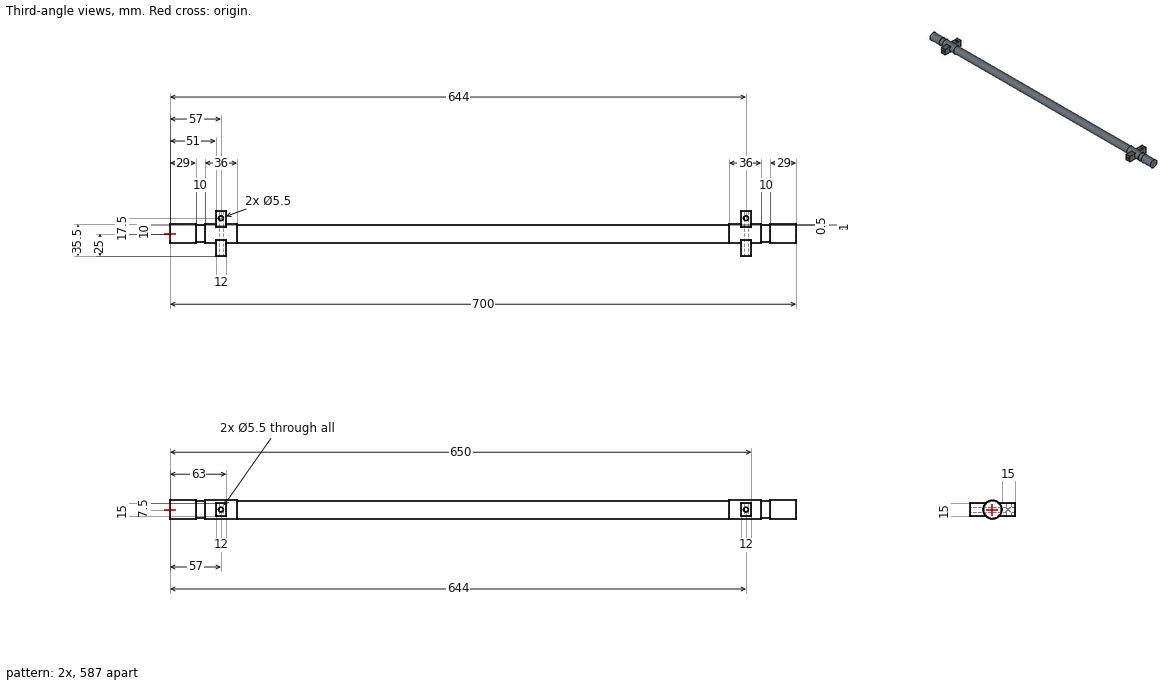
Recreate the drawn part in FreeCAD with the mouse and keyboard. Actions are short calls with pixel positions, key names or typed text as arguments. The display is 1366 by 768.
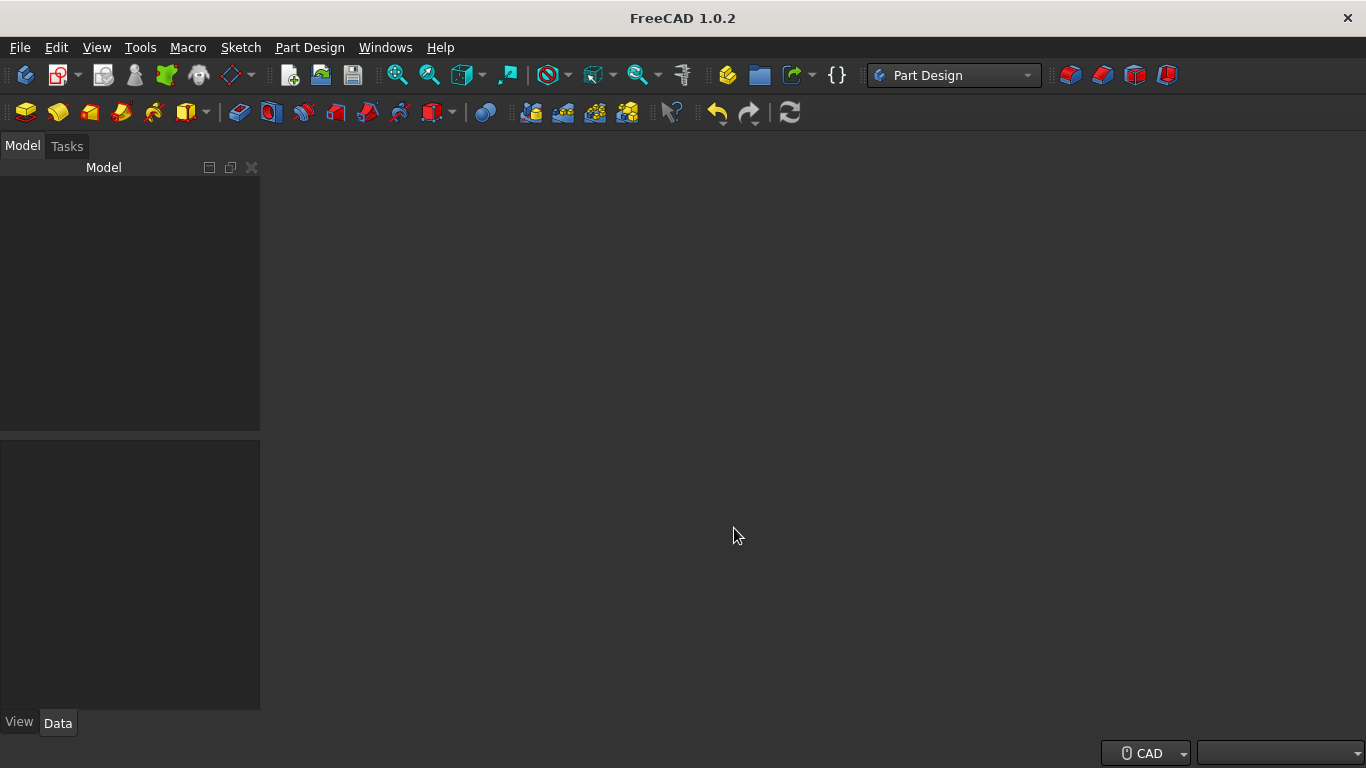
click(290, 76)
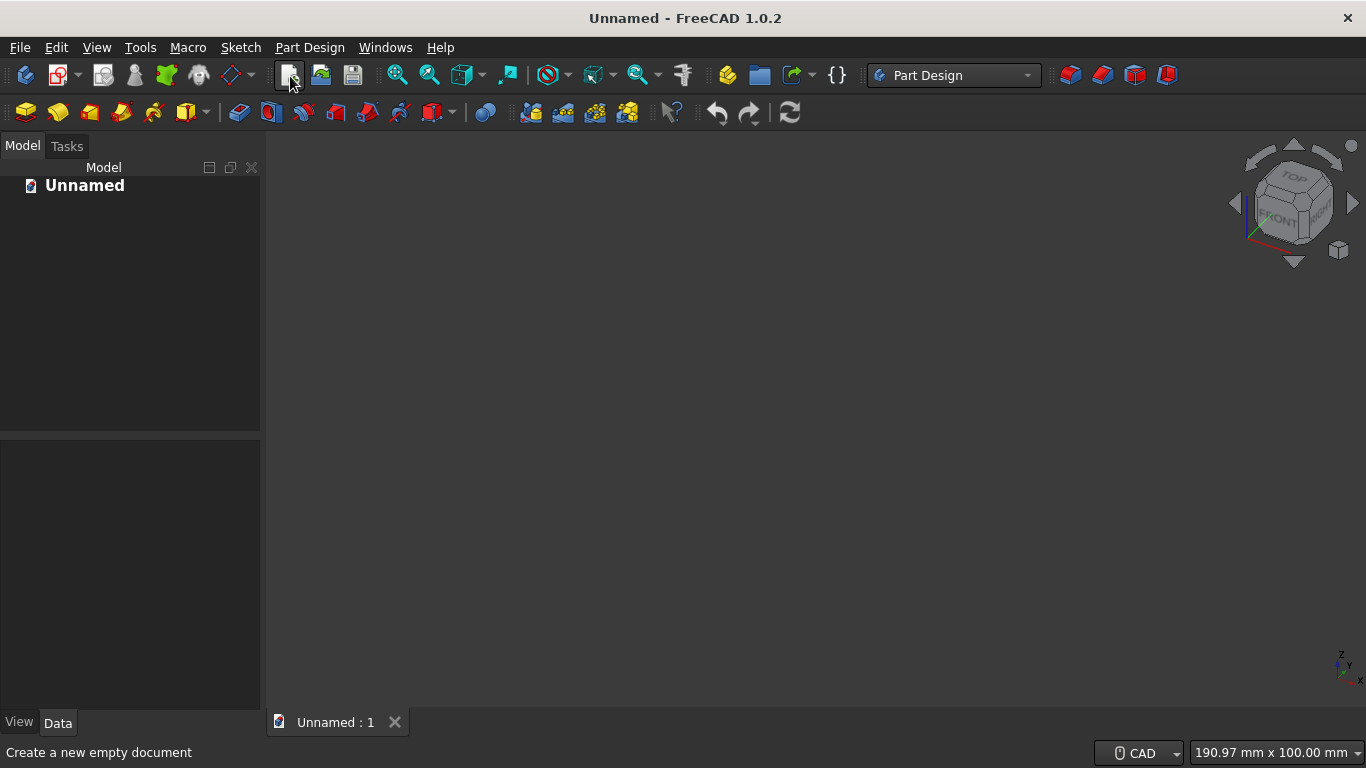
click(58, 76)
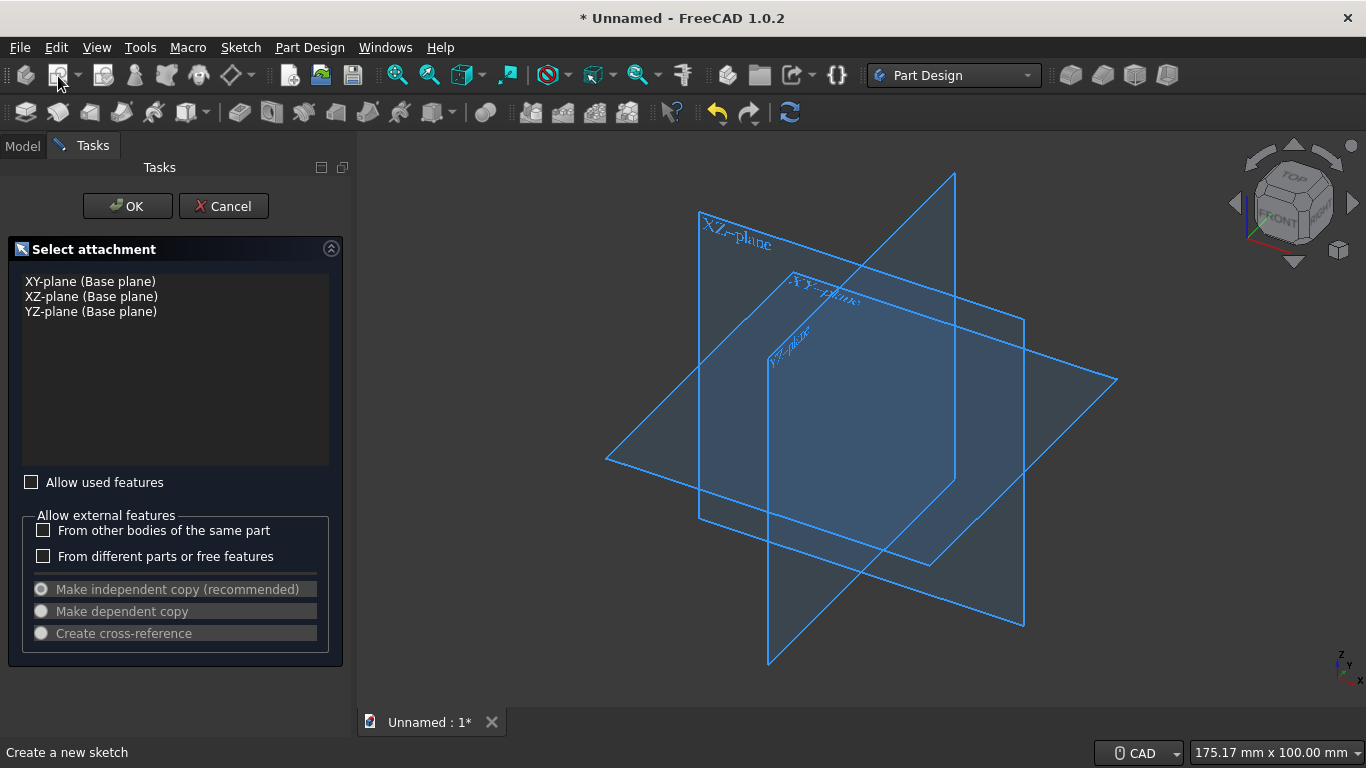
click(82, 282)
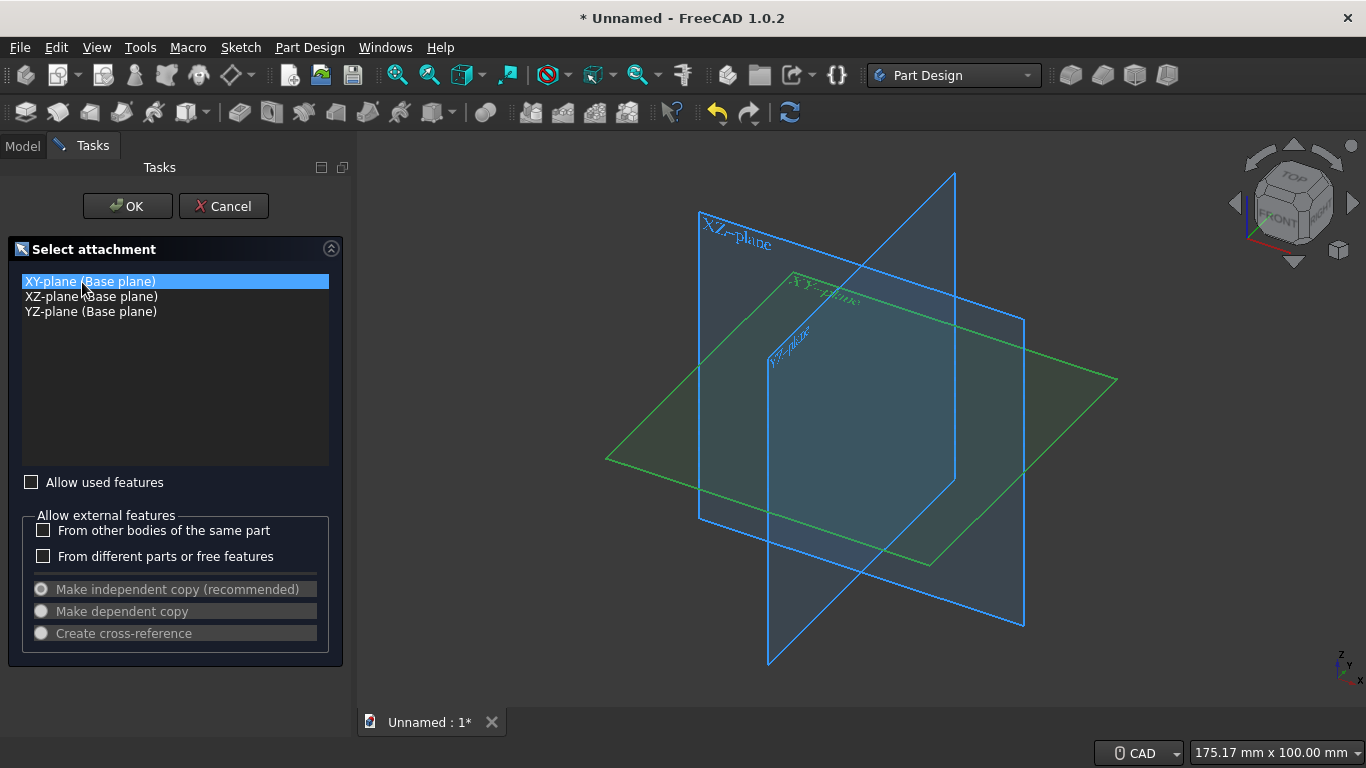
click(128, 206)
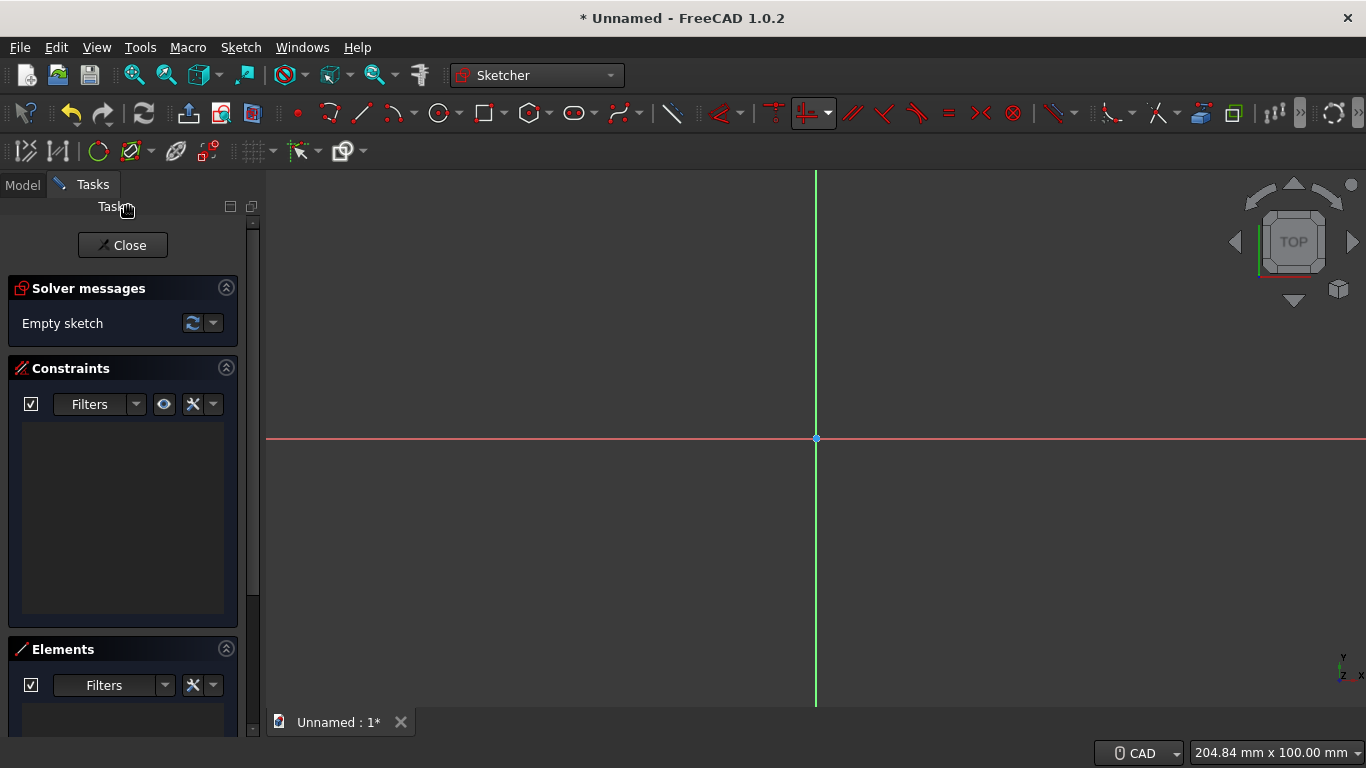
scroll(362, 444, down, 9)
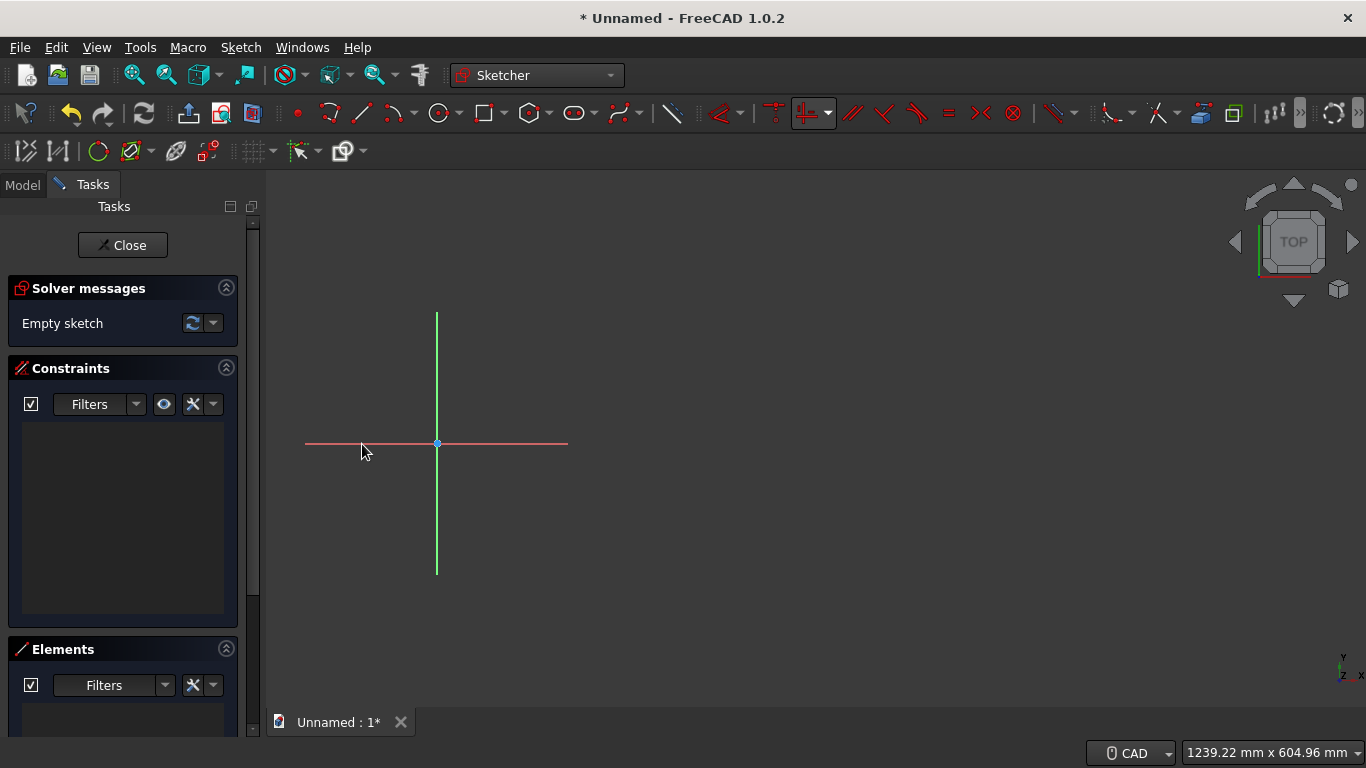
key(g)
key(m)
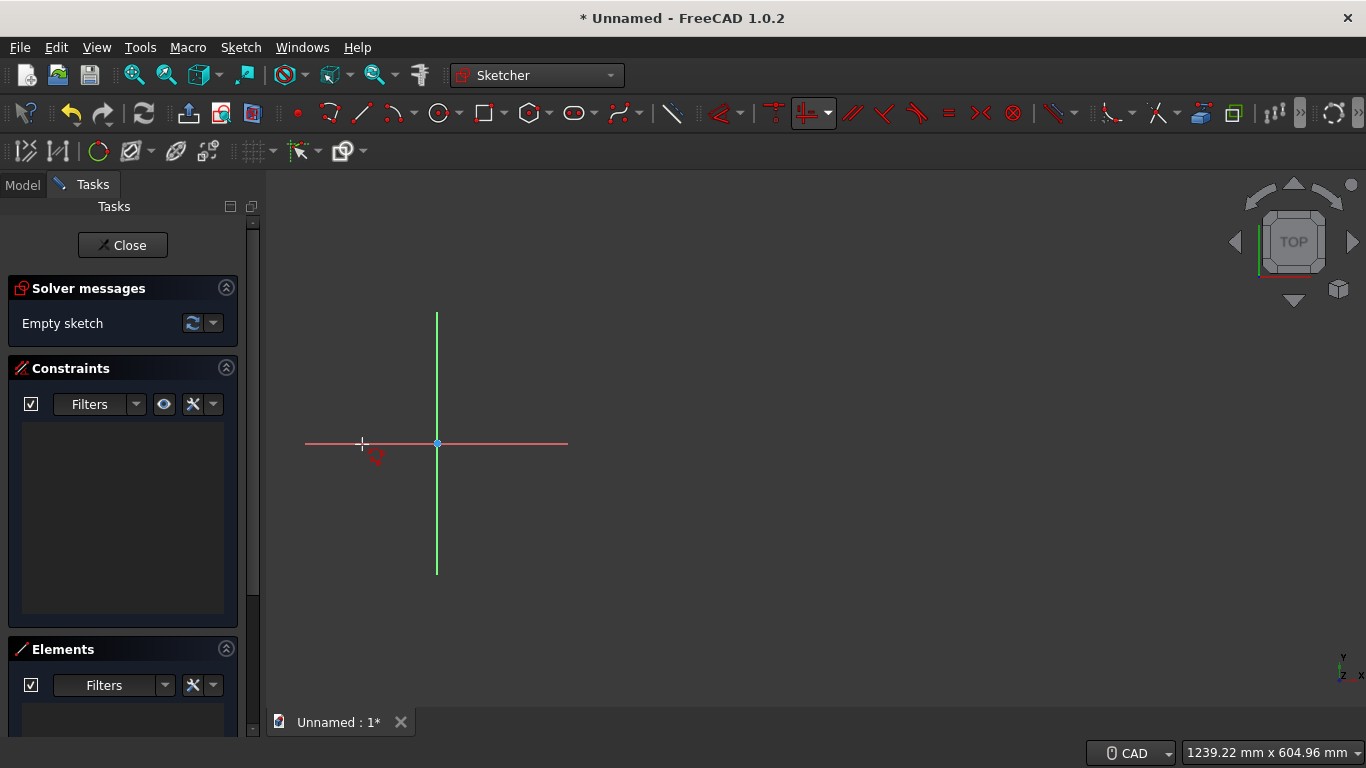
click(437, 444)
click(1058, 435)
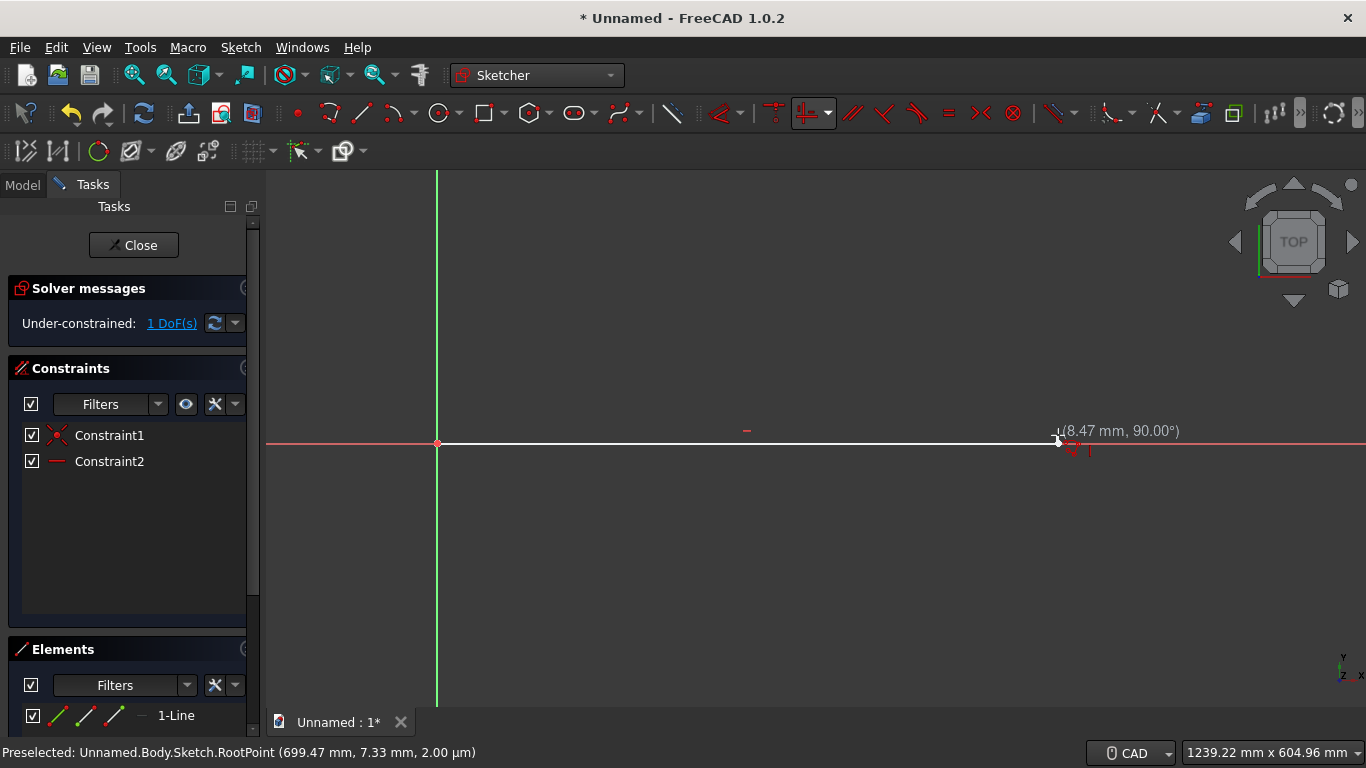
scroll(1058, 434, up, 3)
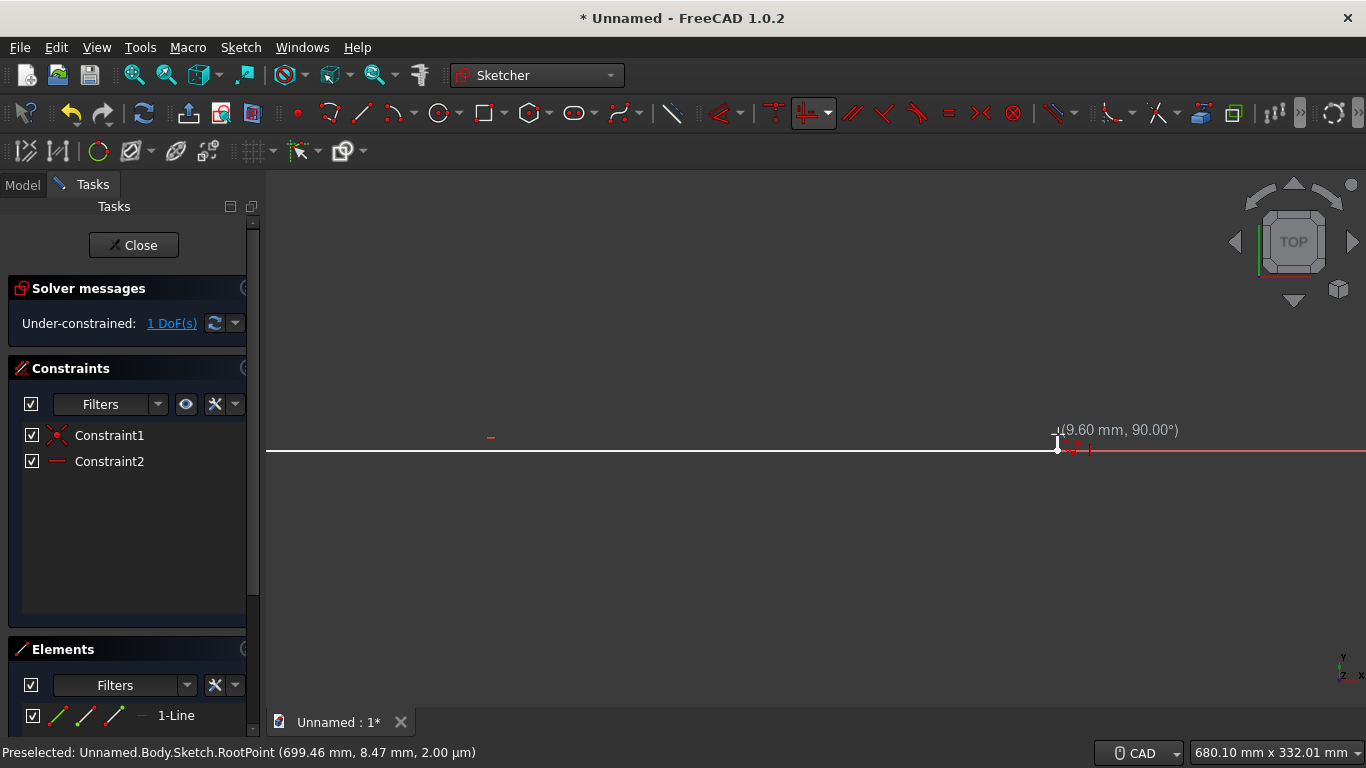
click(1057, 434)
click(1011, 434)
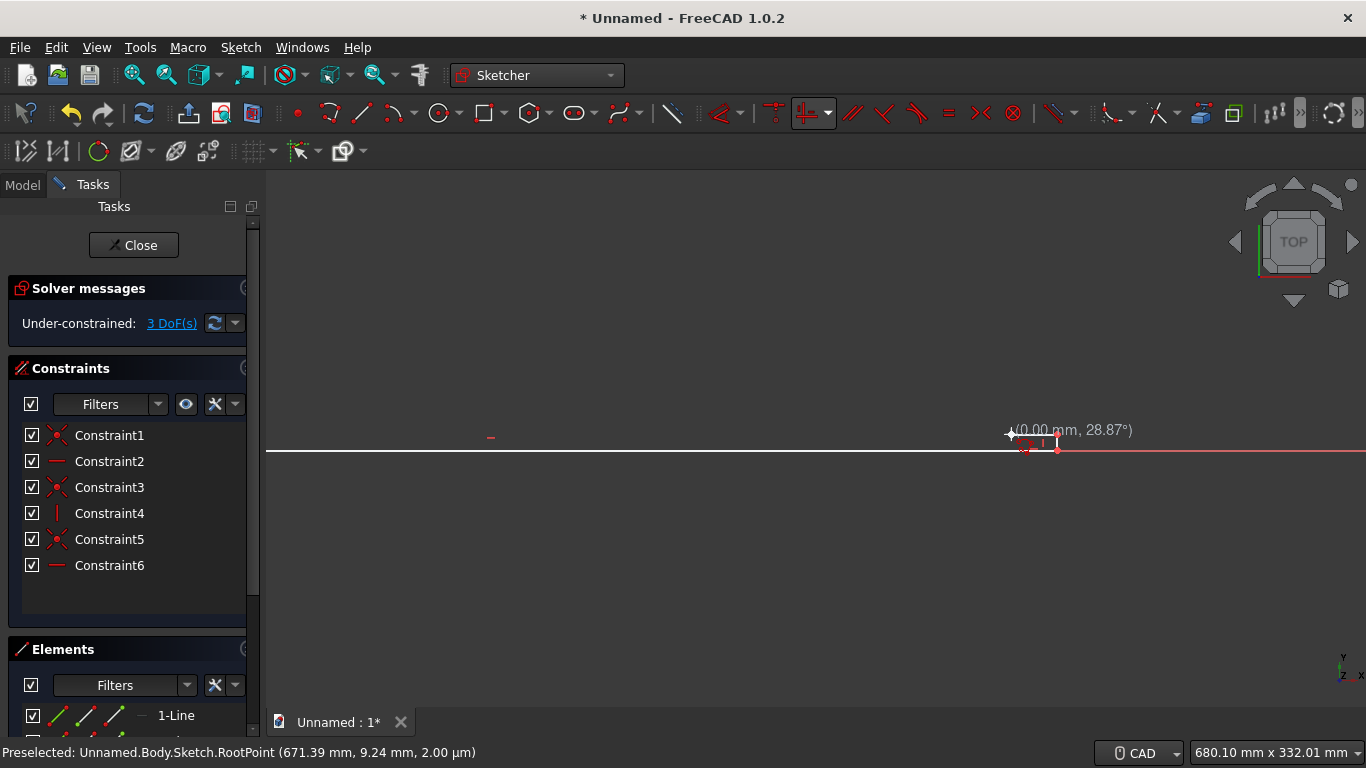
scroll(1011, 436, up, 12)